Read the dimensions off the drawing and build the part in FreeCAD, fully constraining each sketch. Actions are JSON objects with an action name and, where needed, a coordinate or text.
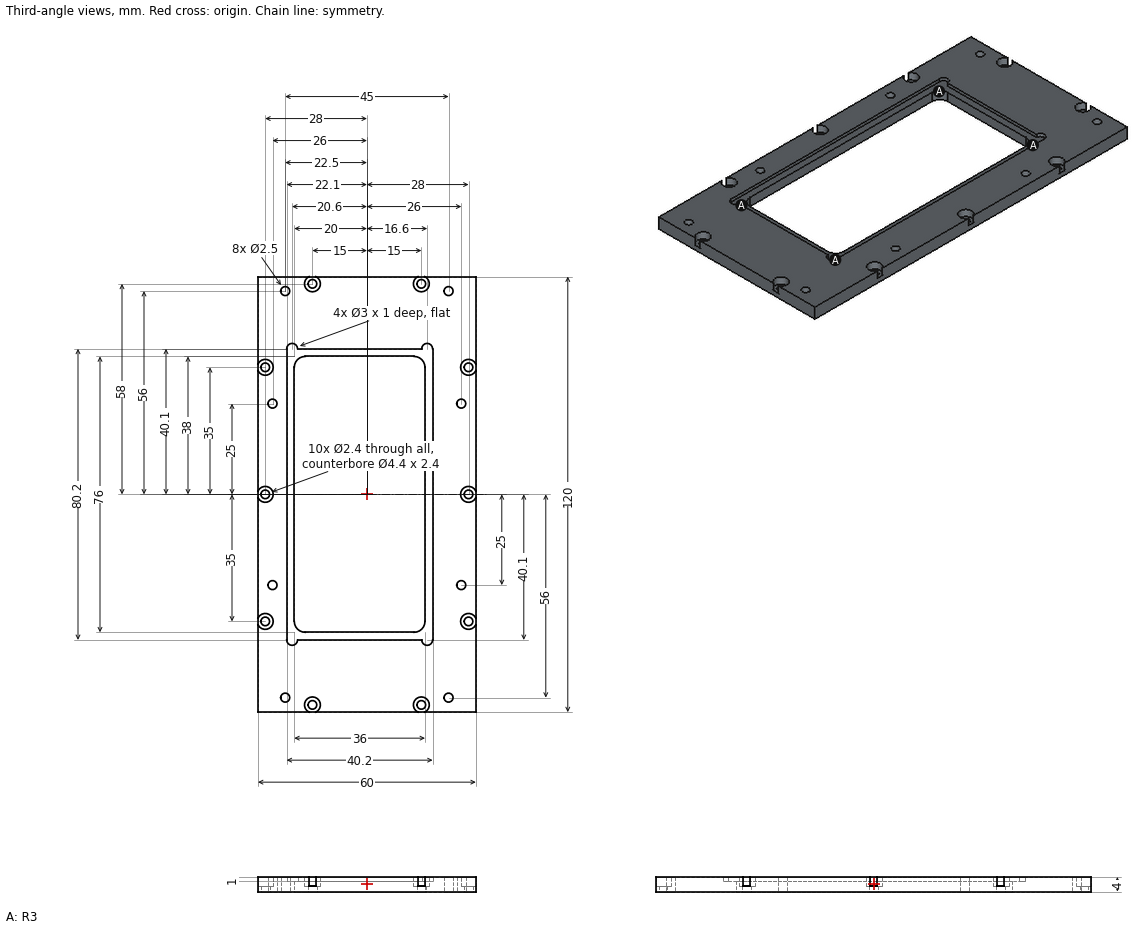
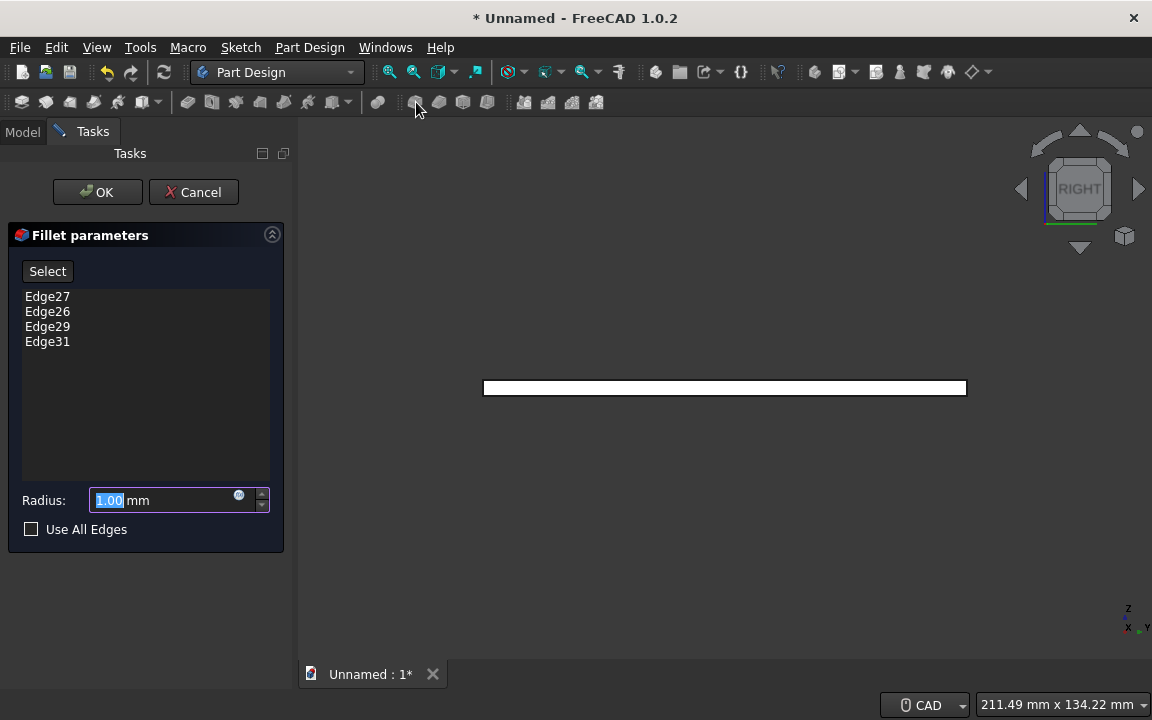
{"action": "type", "text": "3"}
{"action": "key", "text": "Tab"}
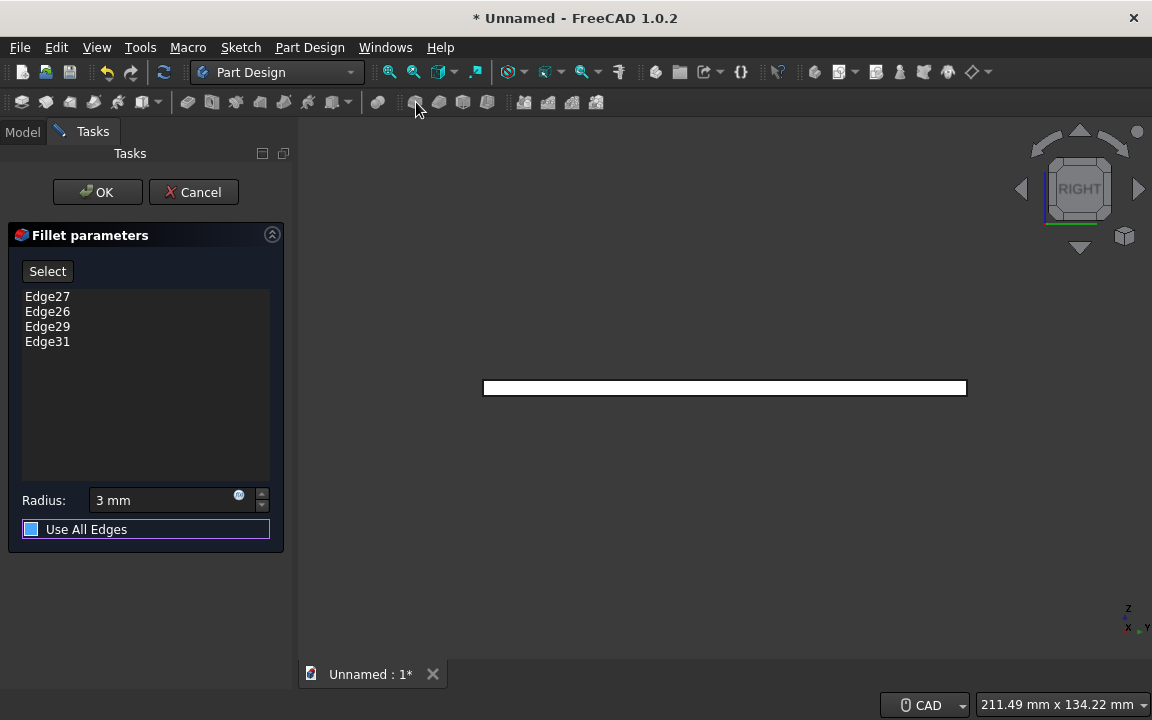
{"action": "left_click", "coordinate": [98, 192]}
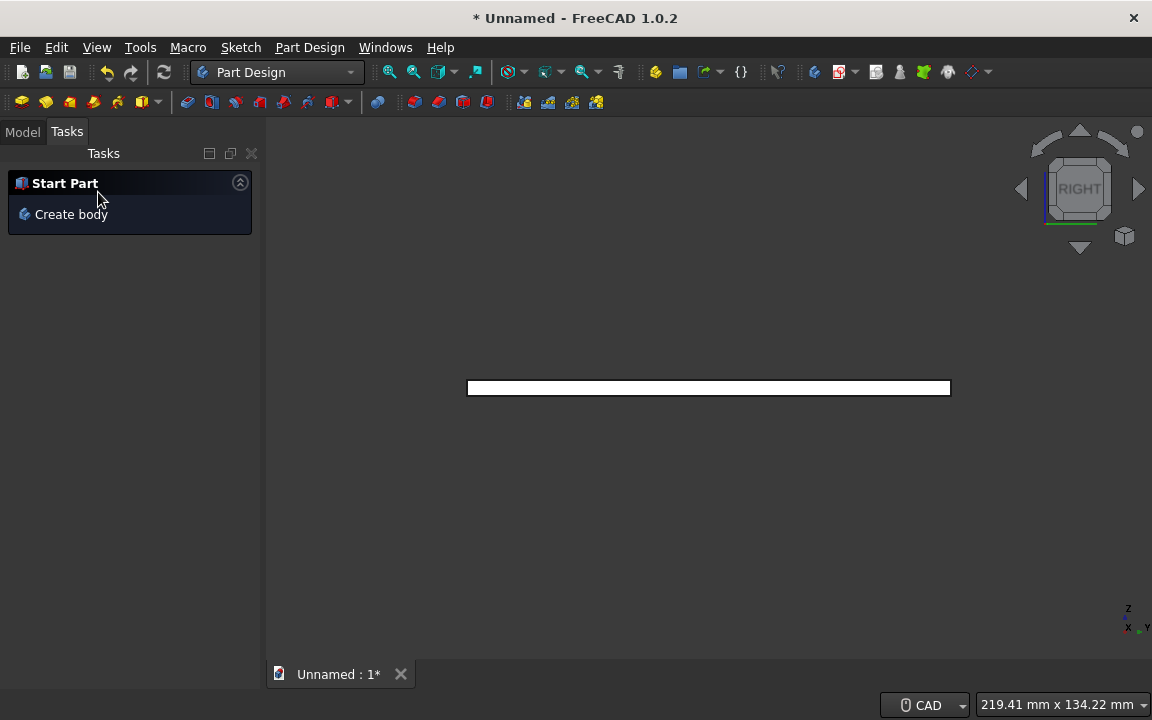
{"action": "key", "text": "0"}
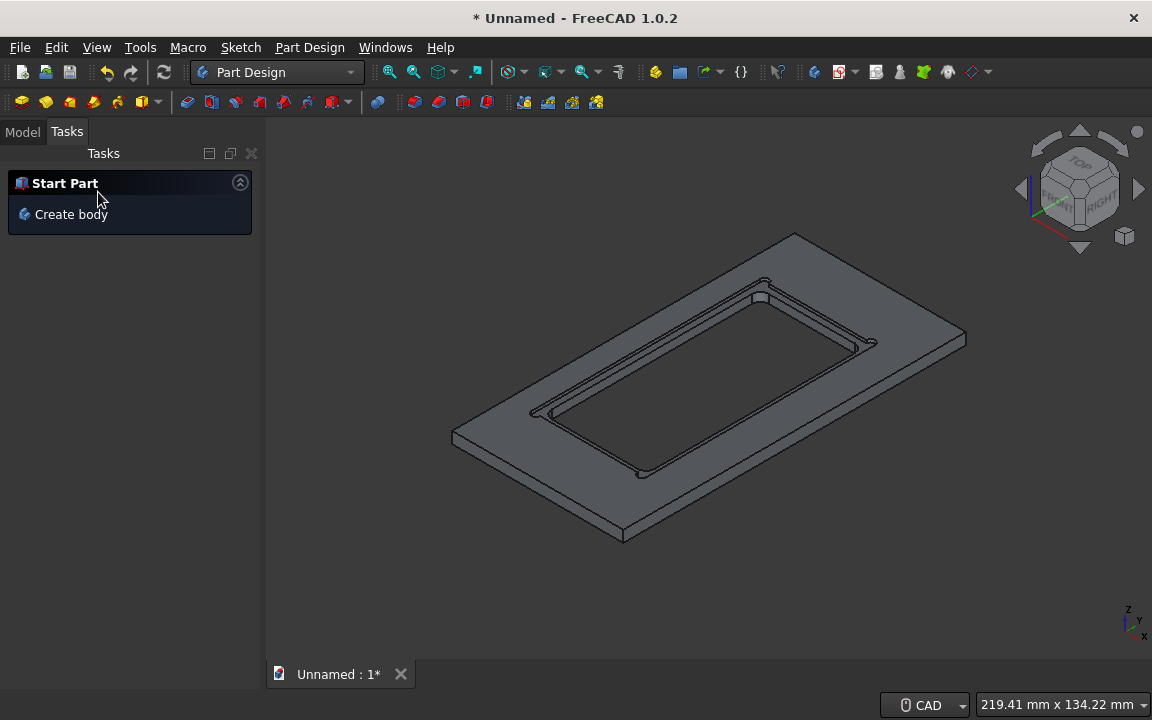
{"action": "left_click", "coordinate": [905, 324]}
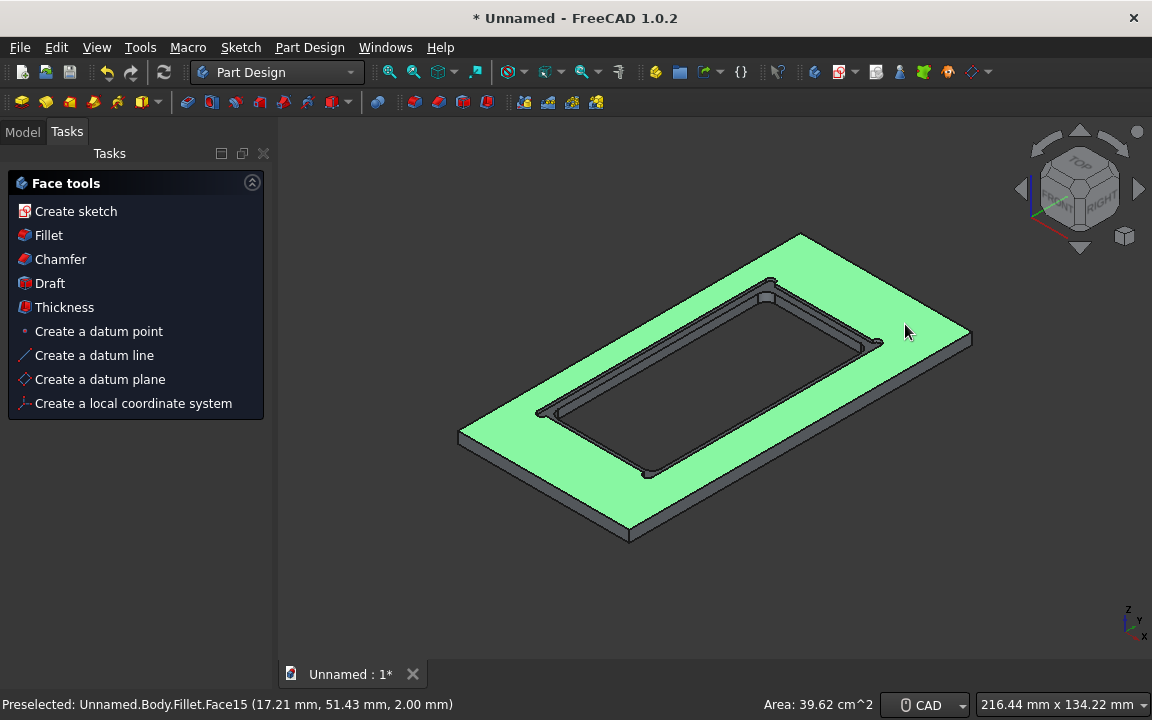
{"action": "left_click", "coordinate": [840, 72]}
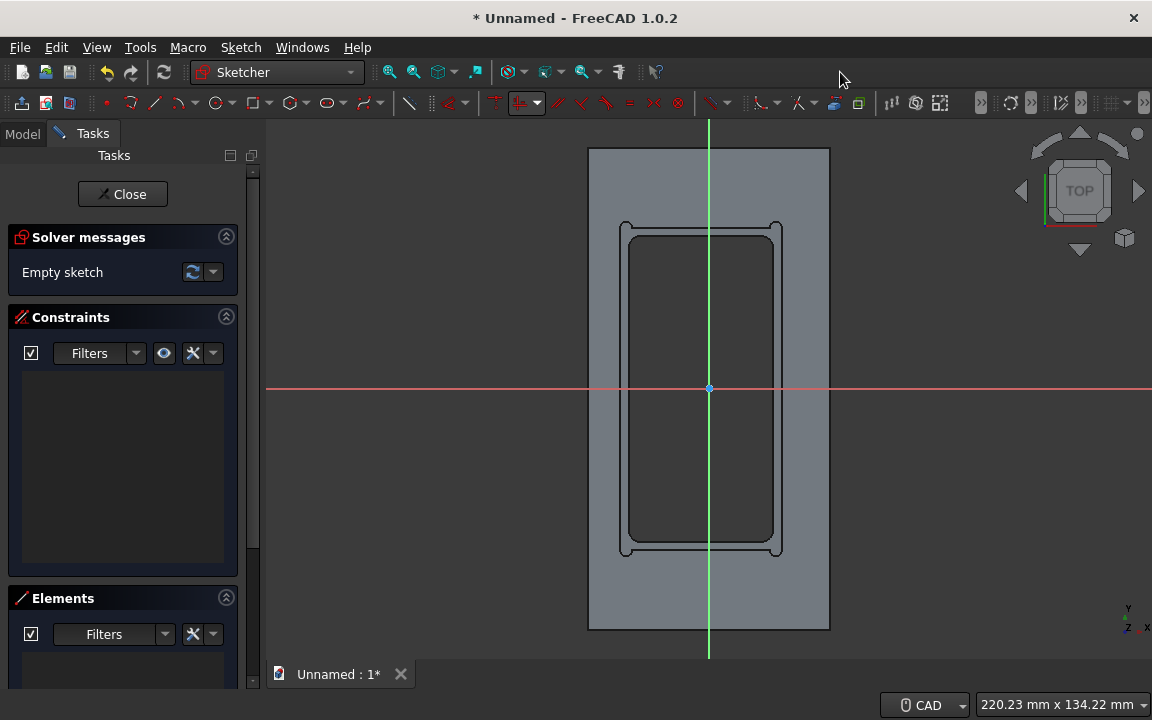
{"action": "scroll", "coordinate": [501, 389], "scroll_direction": "down", "scroll_amount": 2}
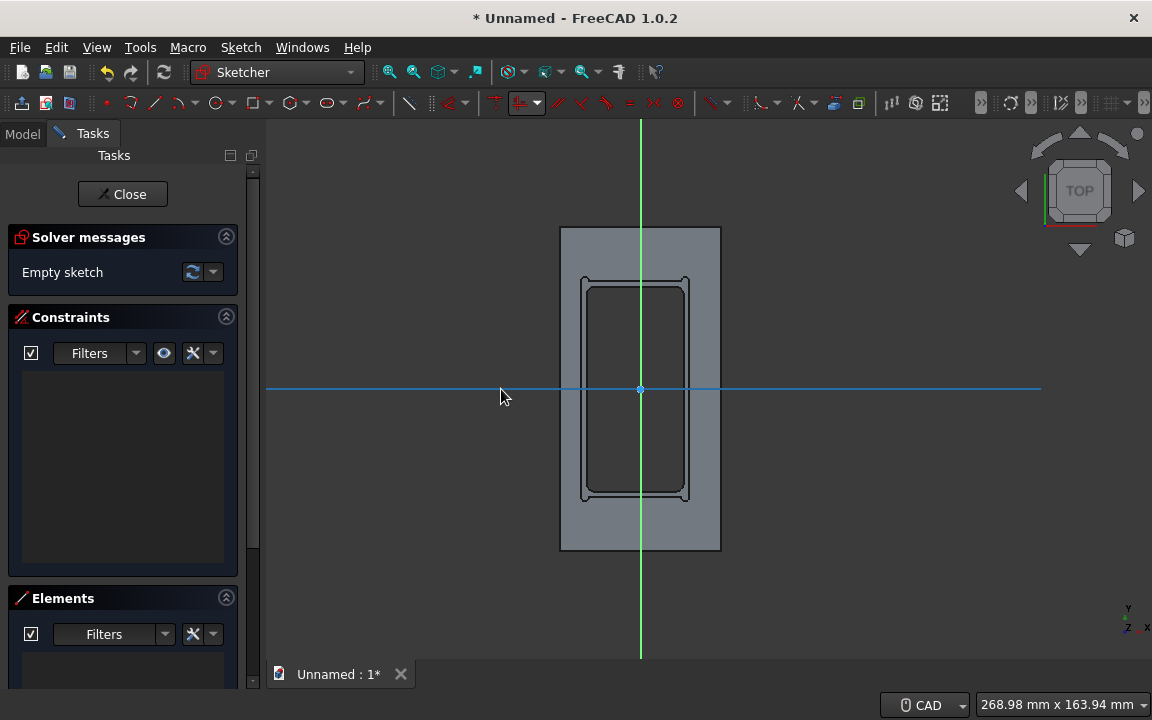
{"action": "key", "text": "g c"}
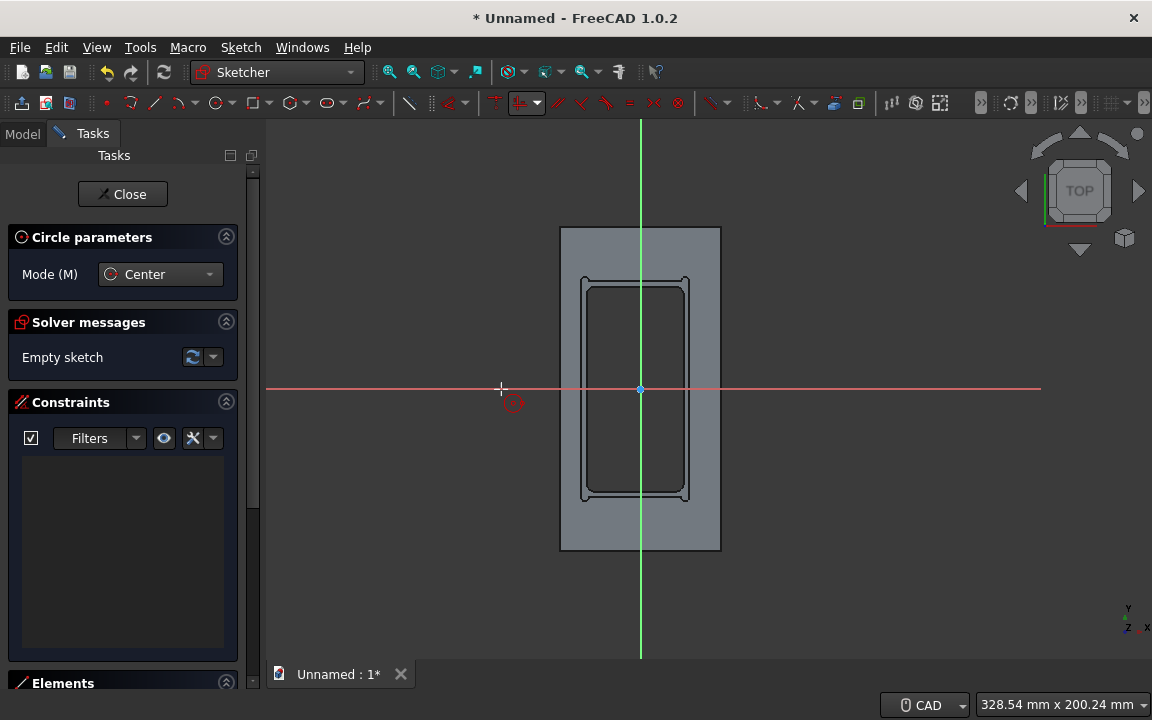
{"action": "scroll", "coordinate": [565, 389], "scroll_direction": "up", "scroll_amount": 10}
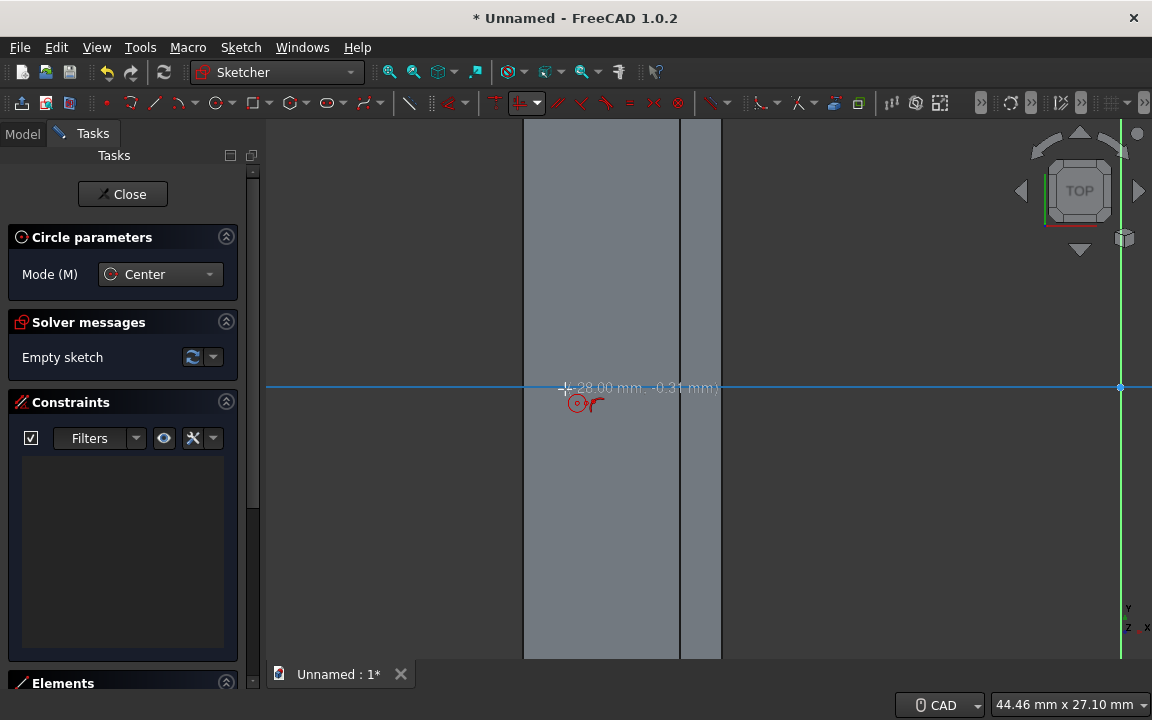
{"action": "scroll", "coordinate": [565, 389], "scroll_direction": "down", "scroll_amount": 10}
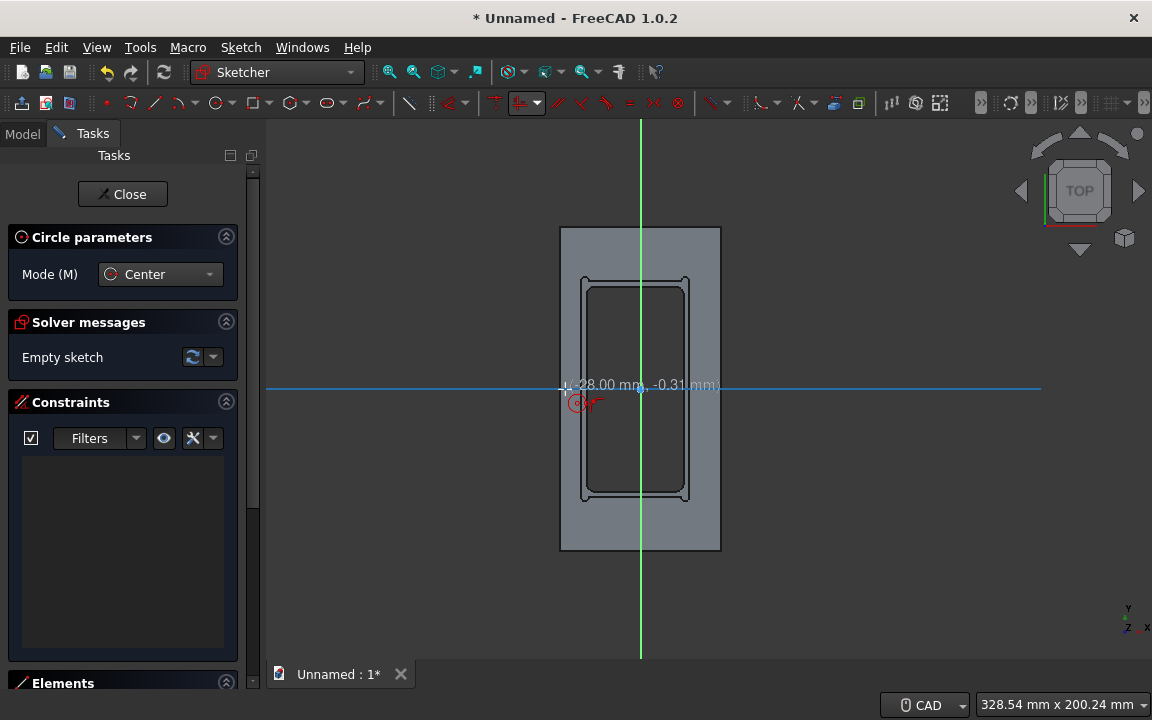
{"action": "left_click", "coordinate": [565, 389]}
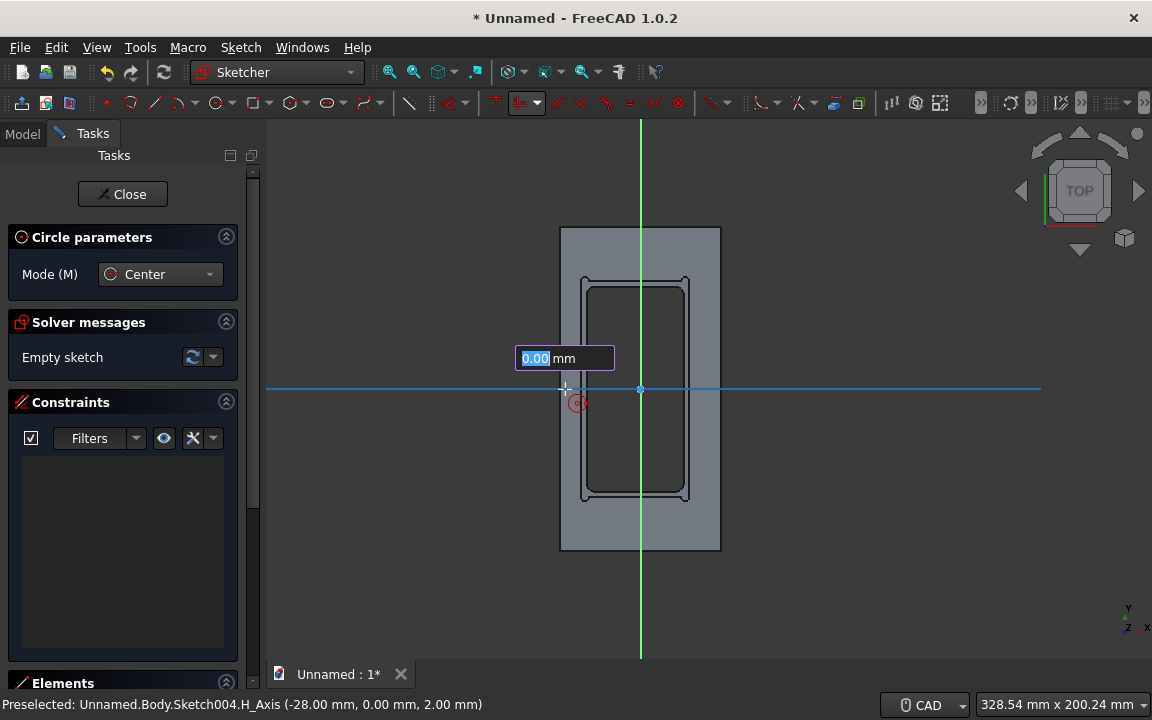
{"action": "scroll", "coordinate": [566, 386], "scroll_direction": "up", "scroll_amount": 9}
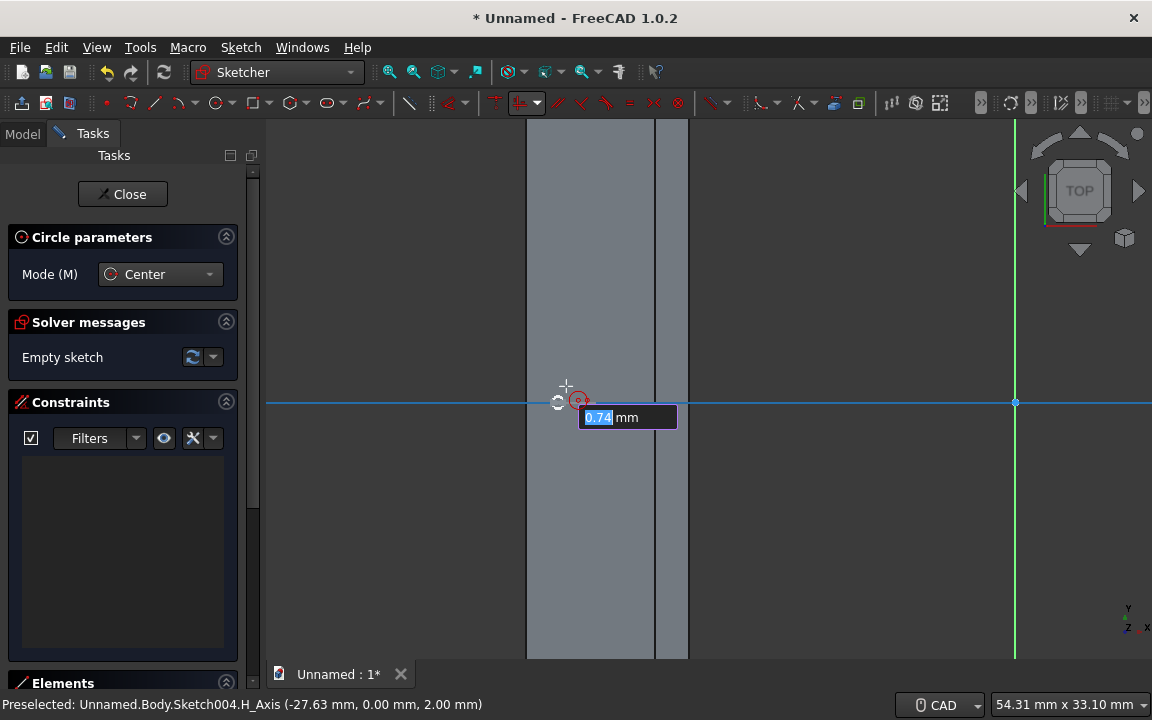
{"action": "left_click", "coordinate": [565, 384]}